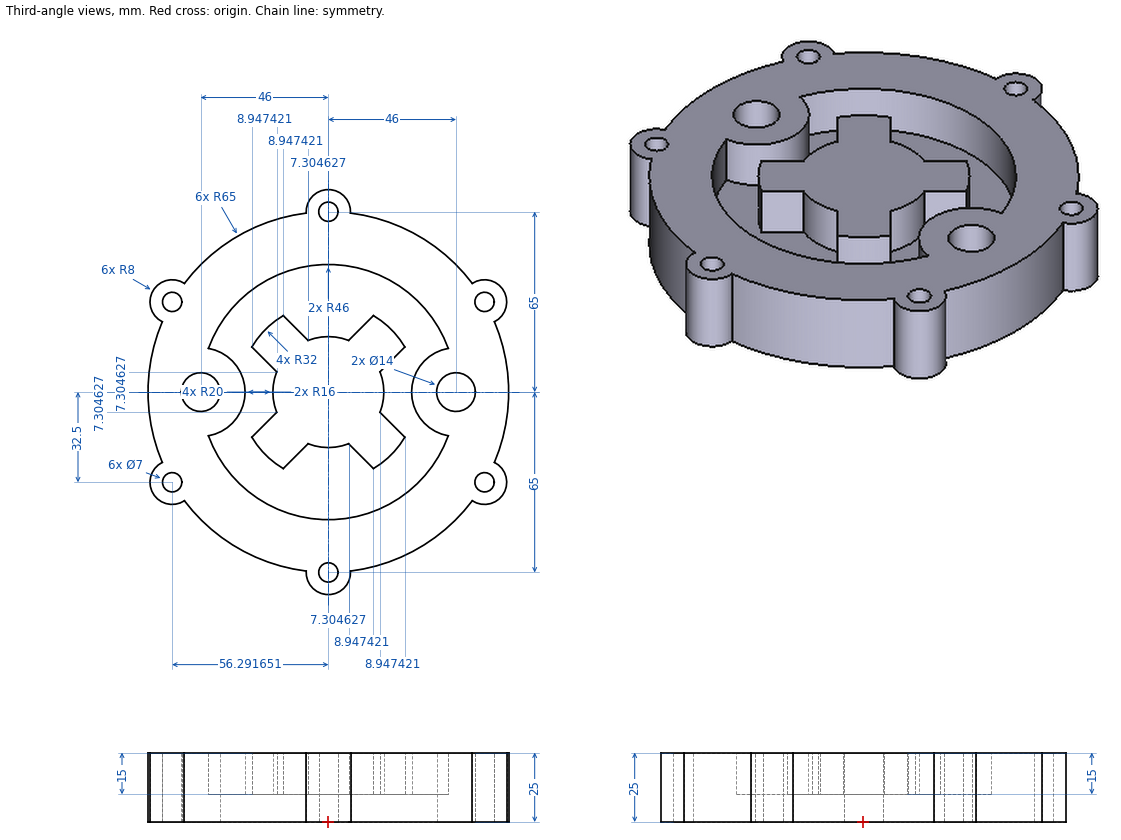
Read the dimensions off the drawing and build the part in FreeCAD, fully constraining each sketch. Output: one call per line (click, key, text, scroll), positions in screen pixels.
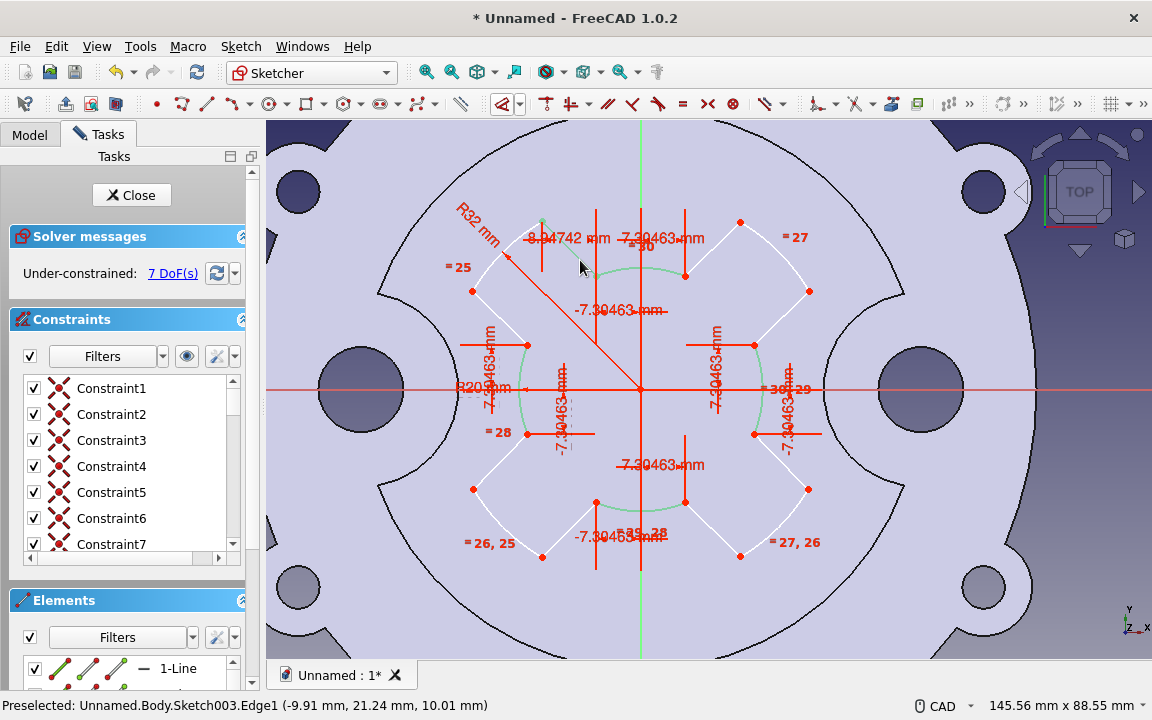
click(489, 307)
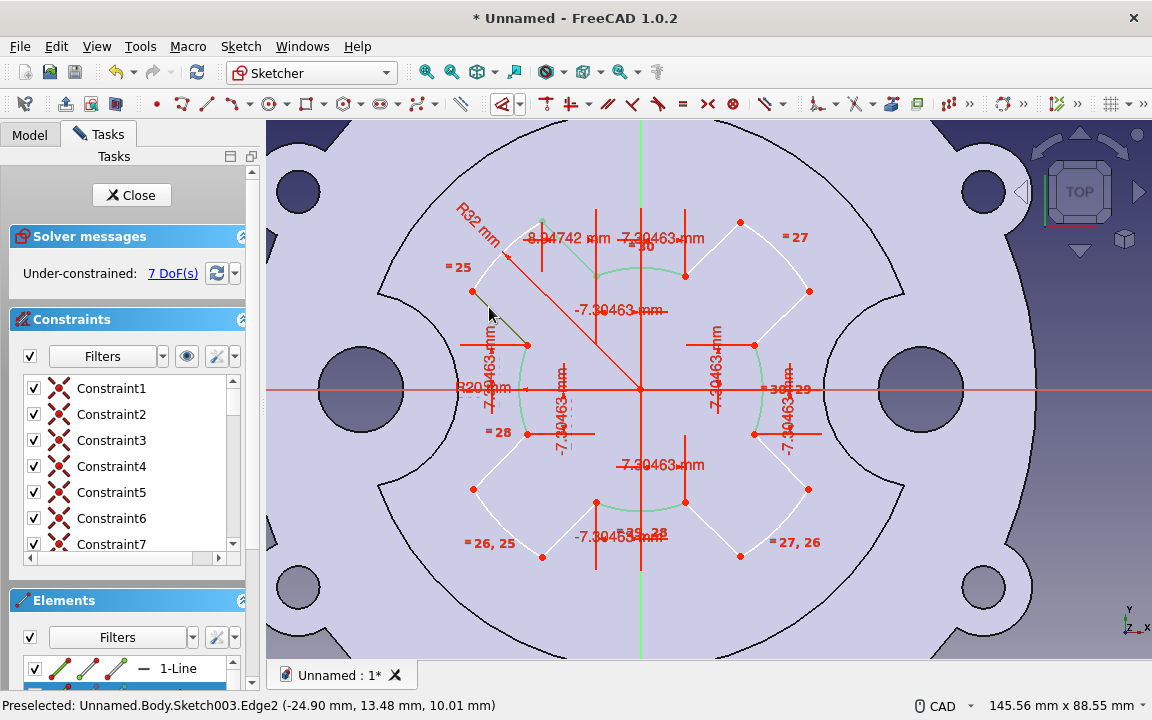
click(520, 104)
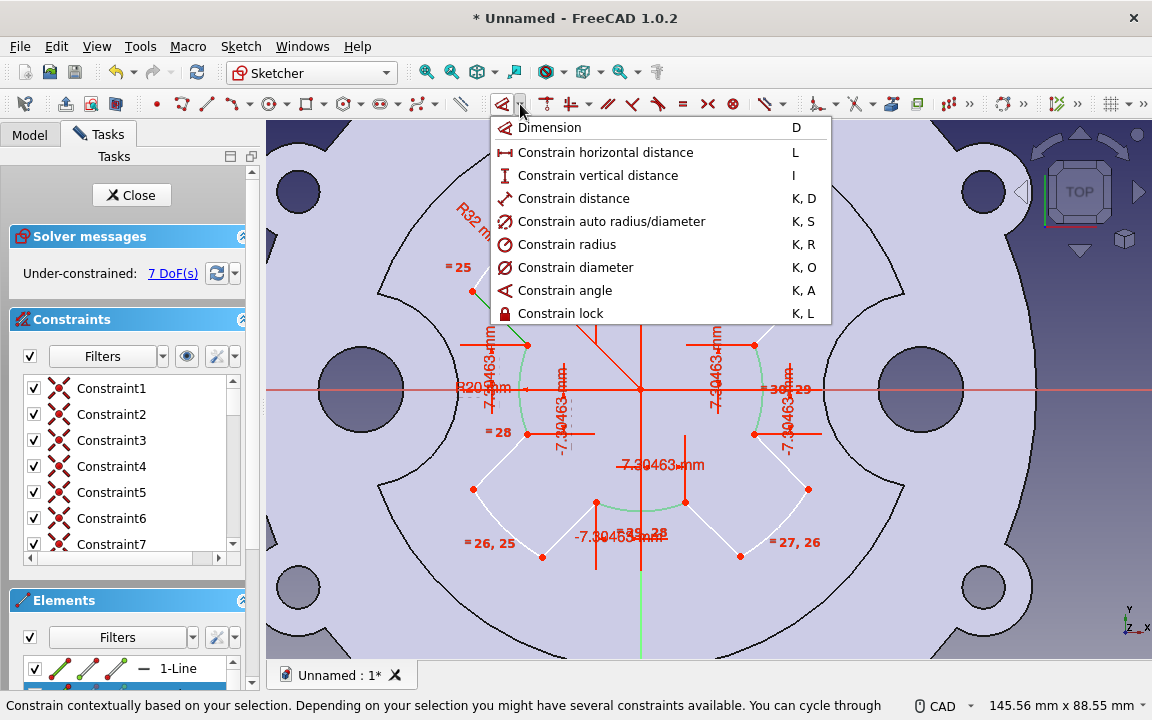
click(661, 152)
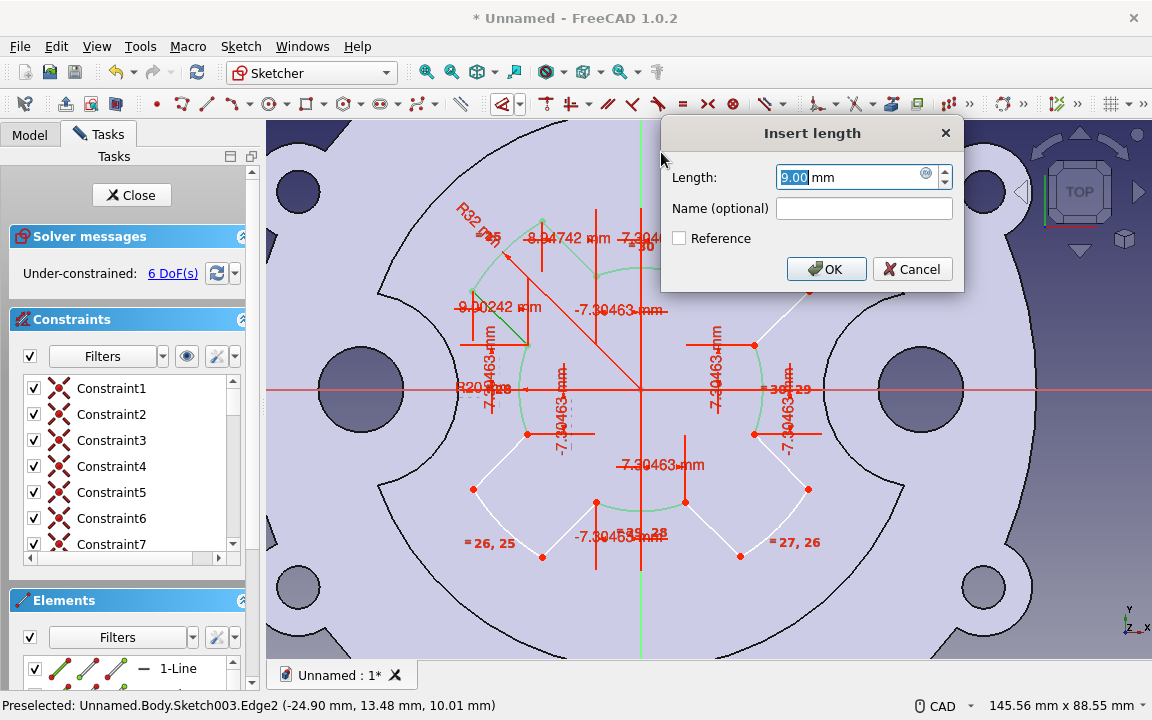
text(8.947421)
key(Return)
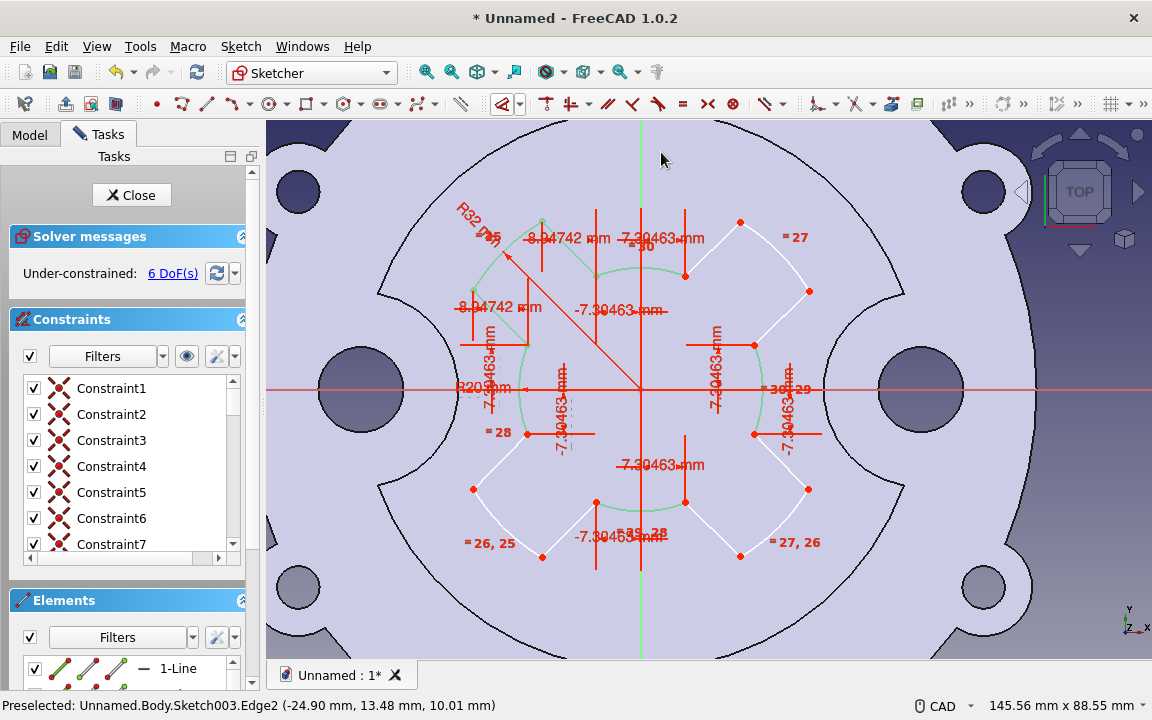
click(511, 451)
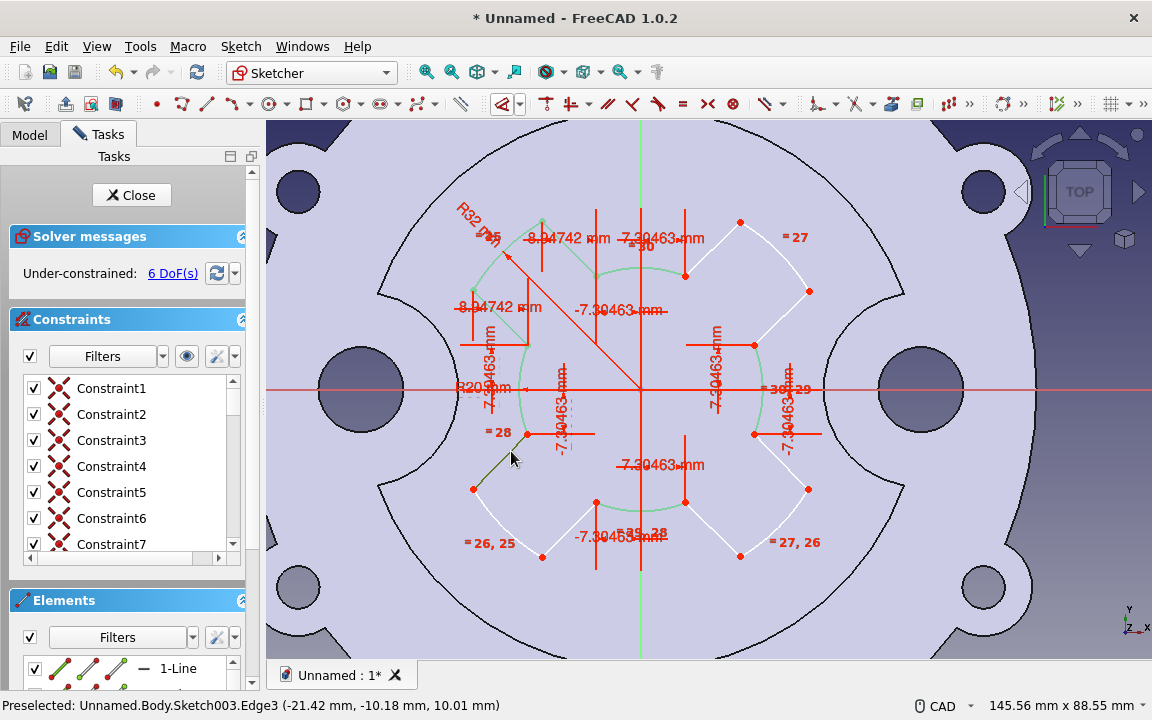
click(520, 104)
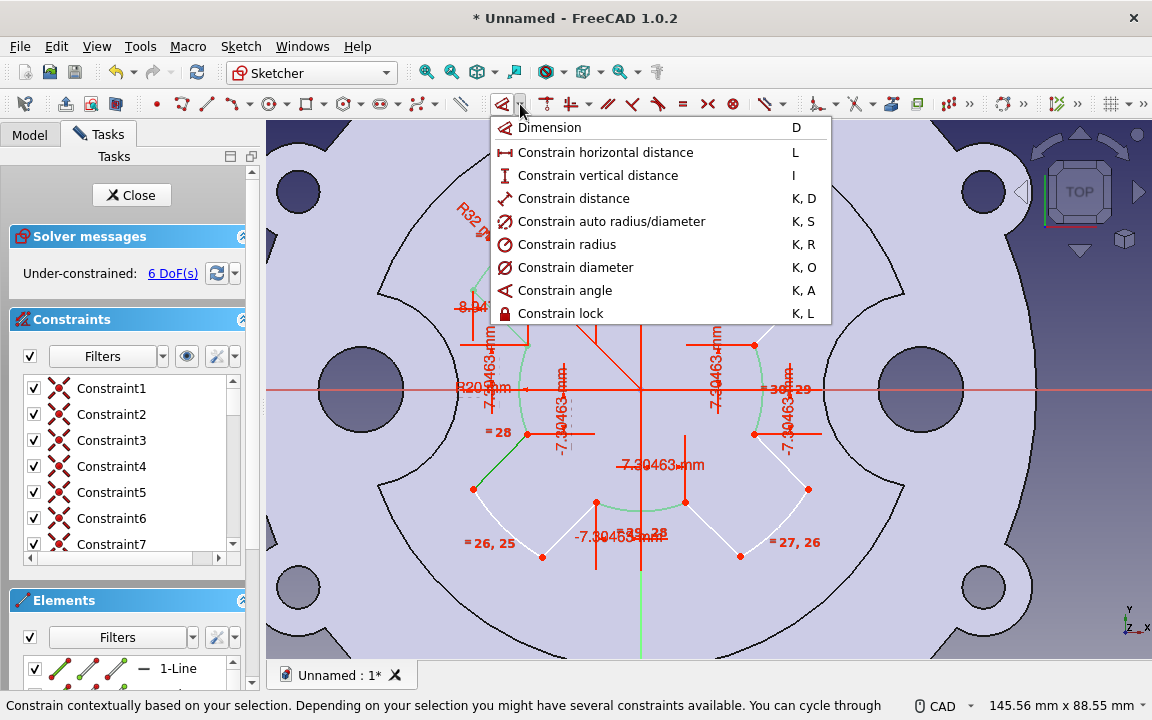
click(661, 152)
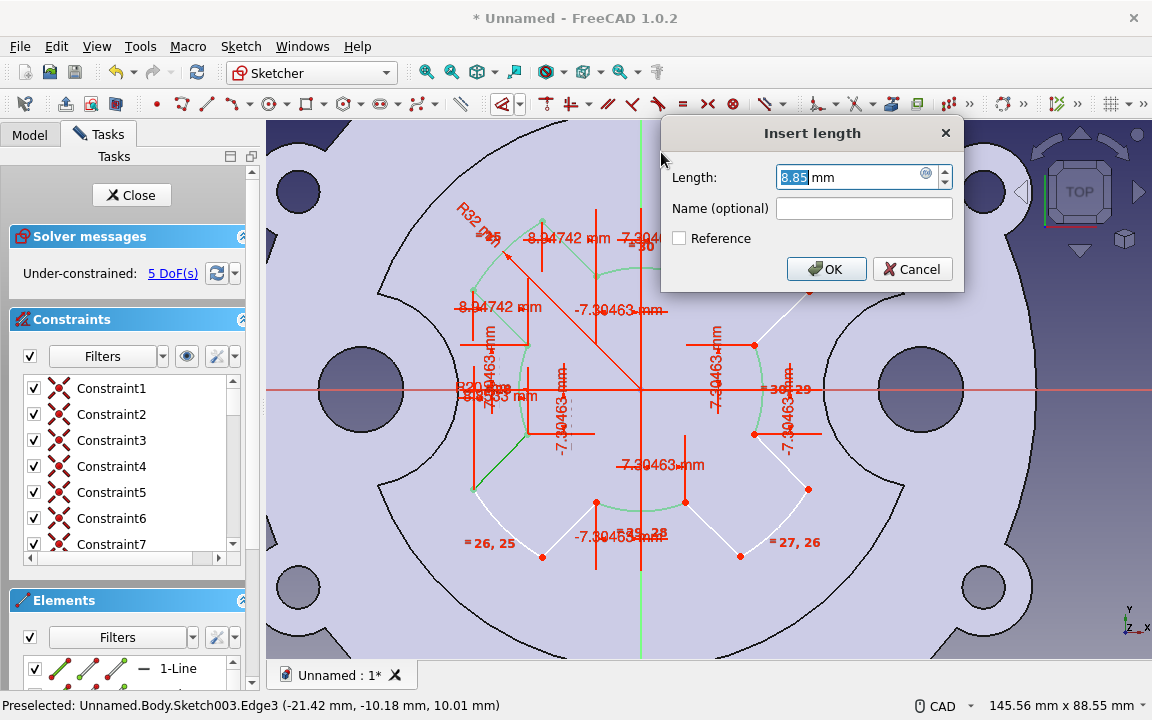
text(8.947421)
key(Return)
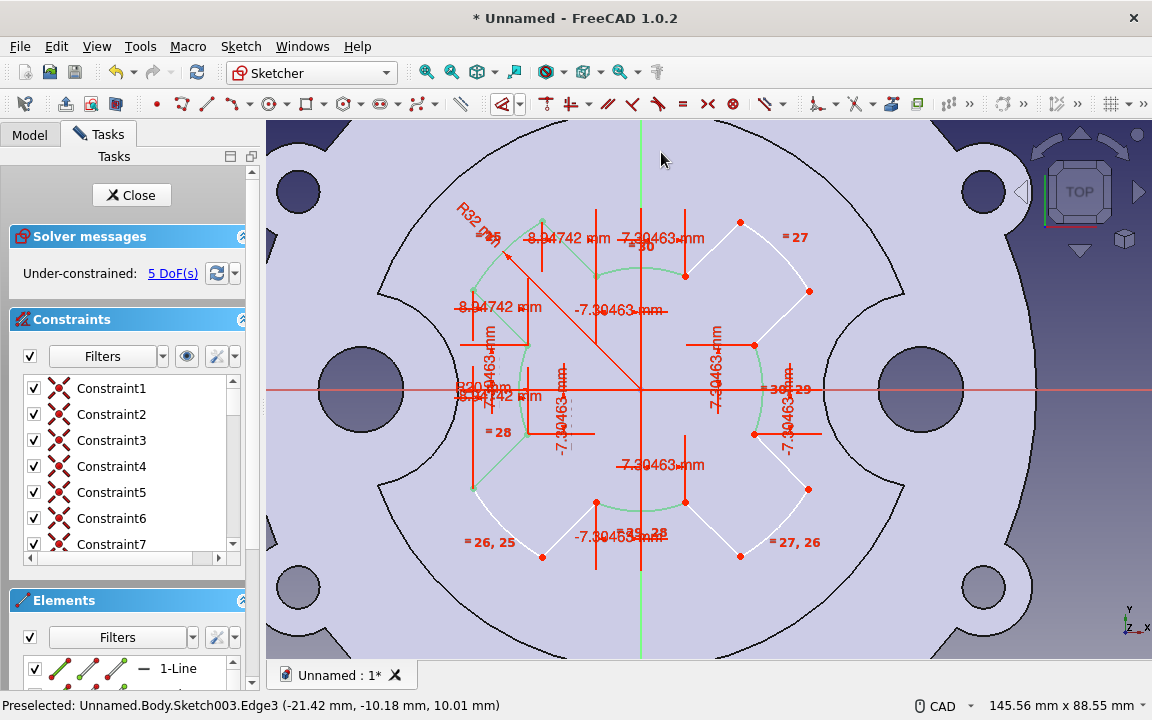
click(558, 541)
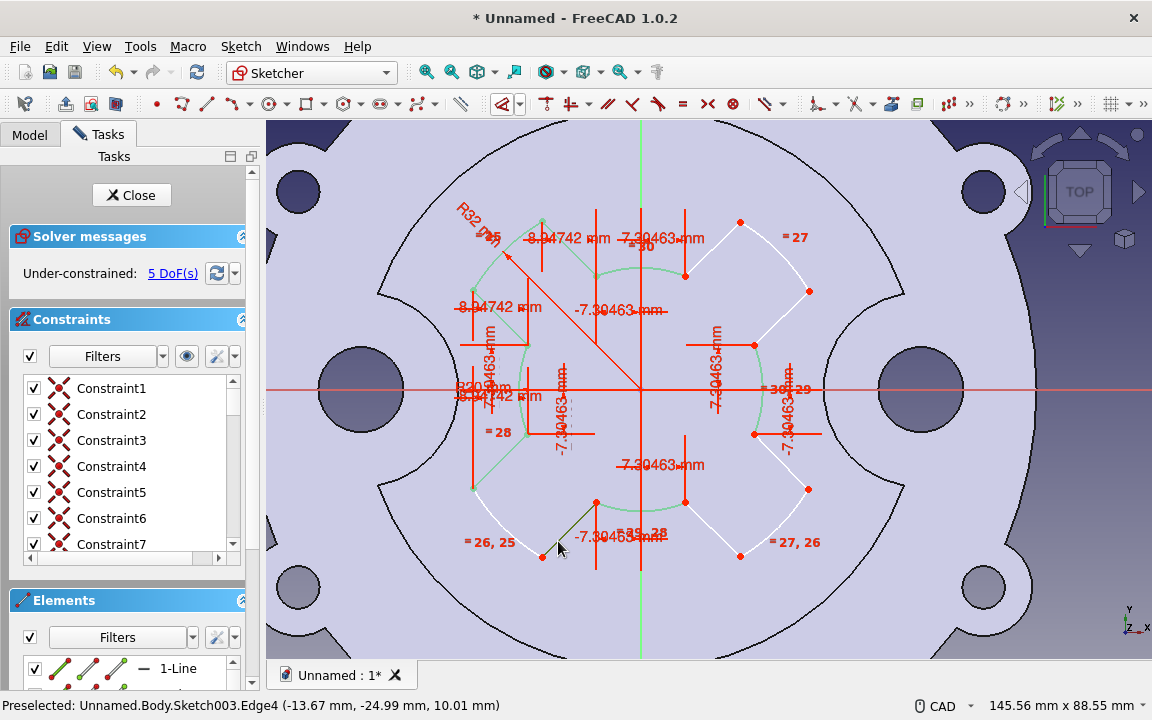
key(l)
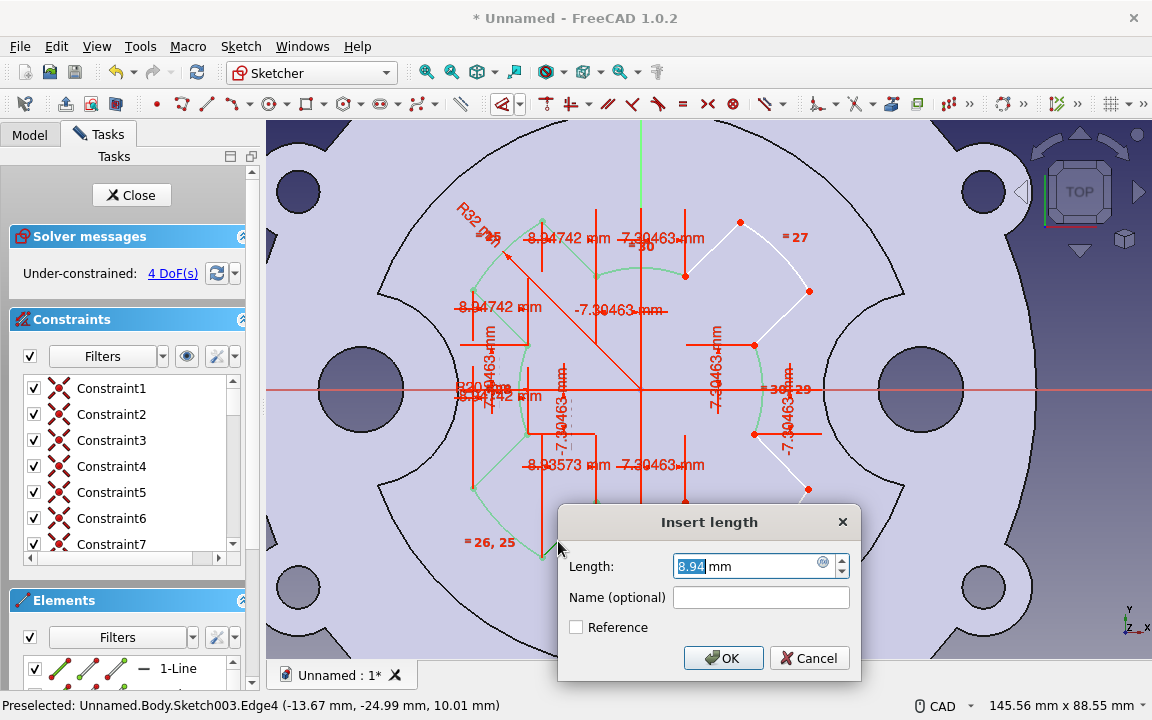
text(8.947421)
key(Return)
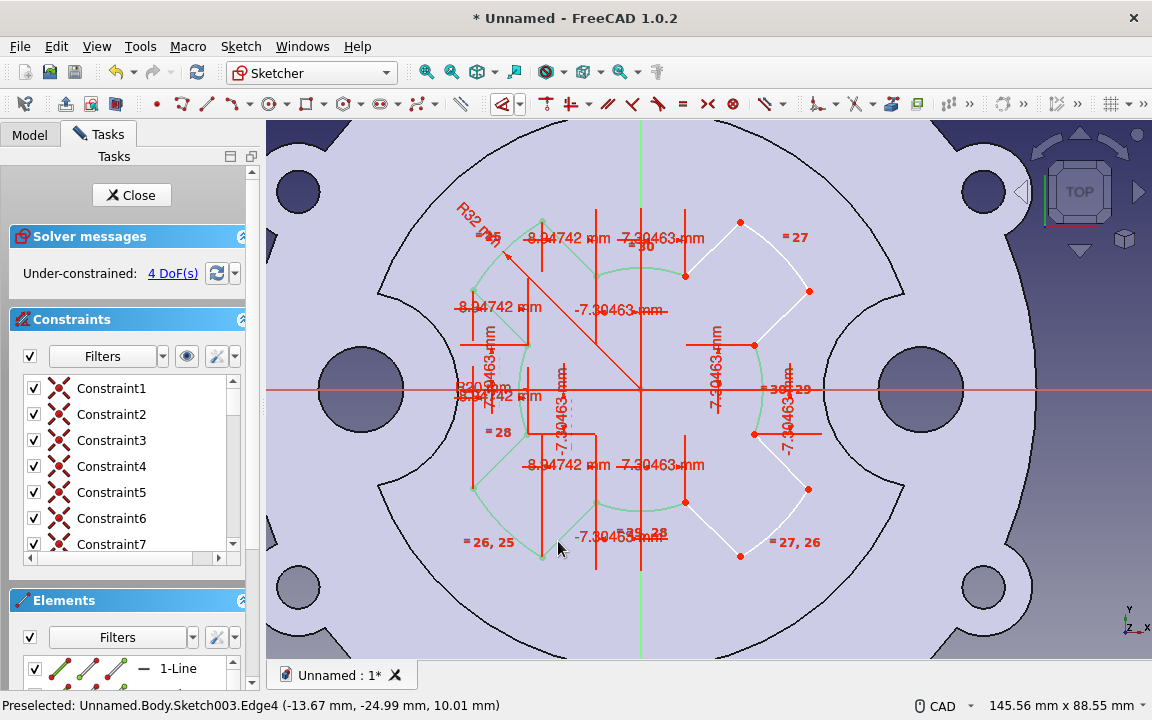
click(702, 519)